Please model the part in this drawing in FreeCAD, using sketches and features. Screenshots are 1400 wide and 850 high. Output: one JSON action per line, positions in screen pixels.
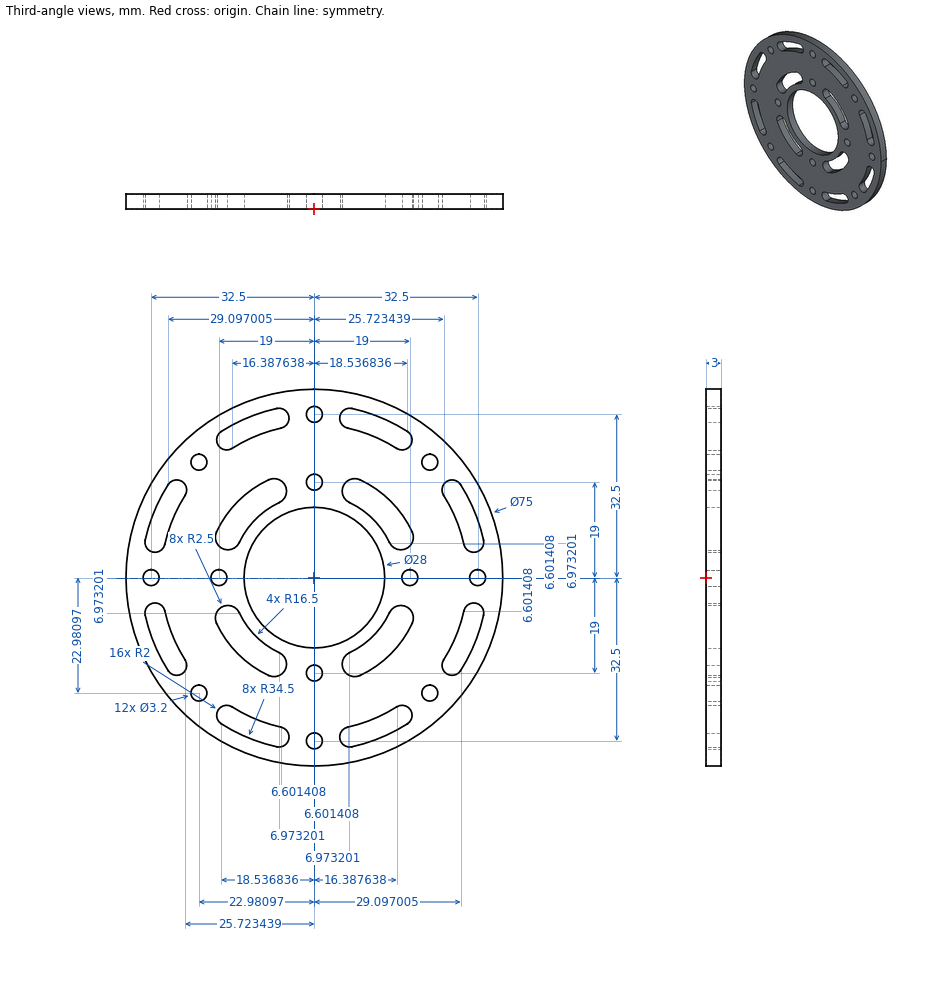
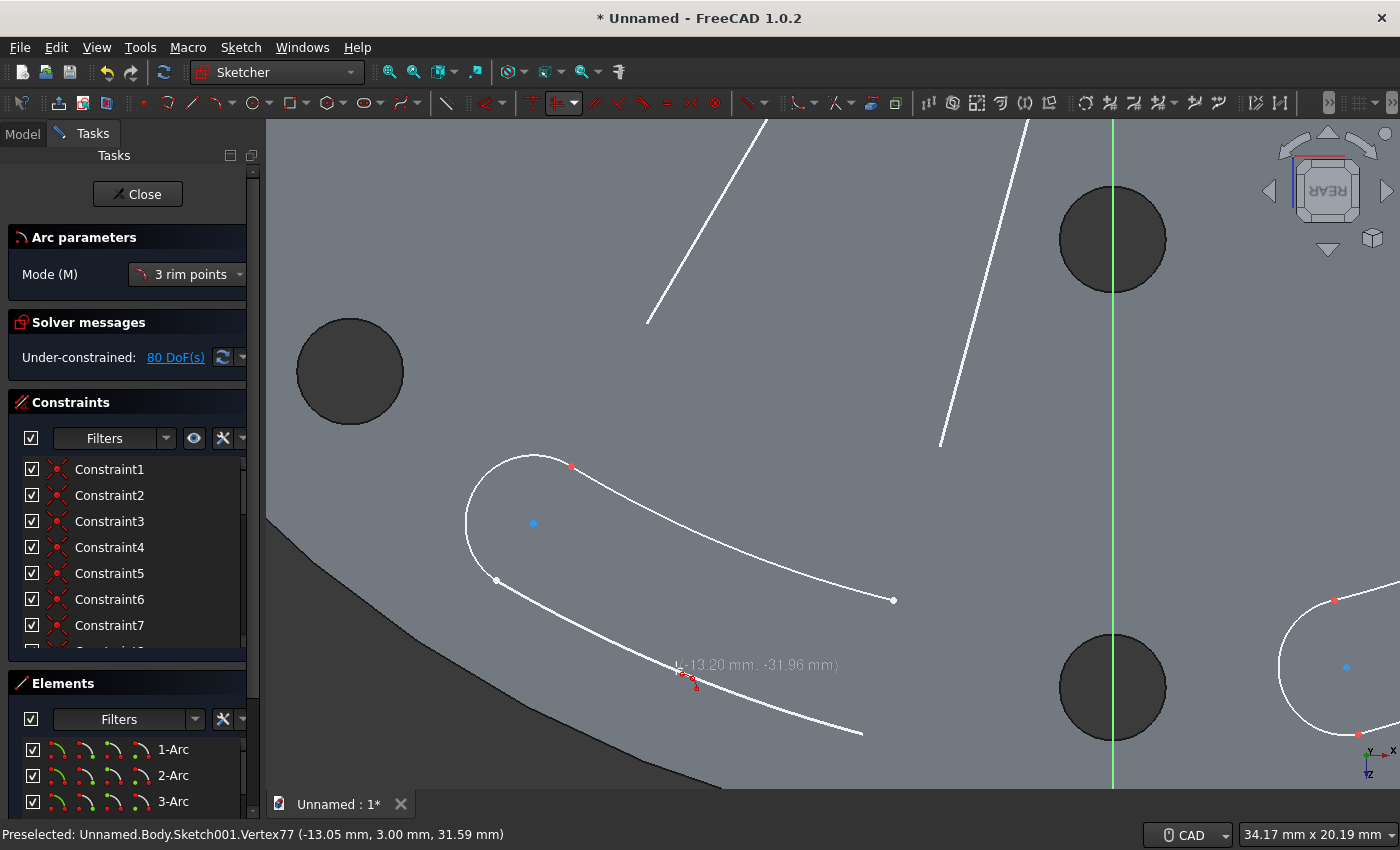
{"action": "left_click", "coordinate": [675, 667]}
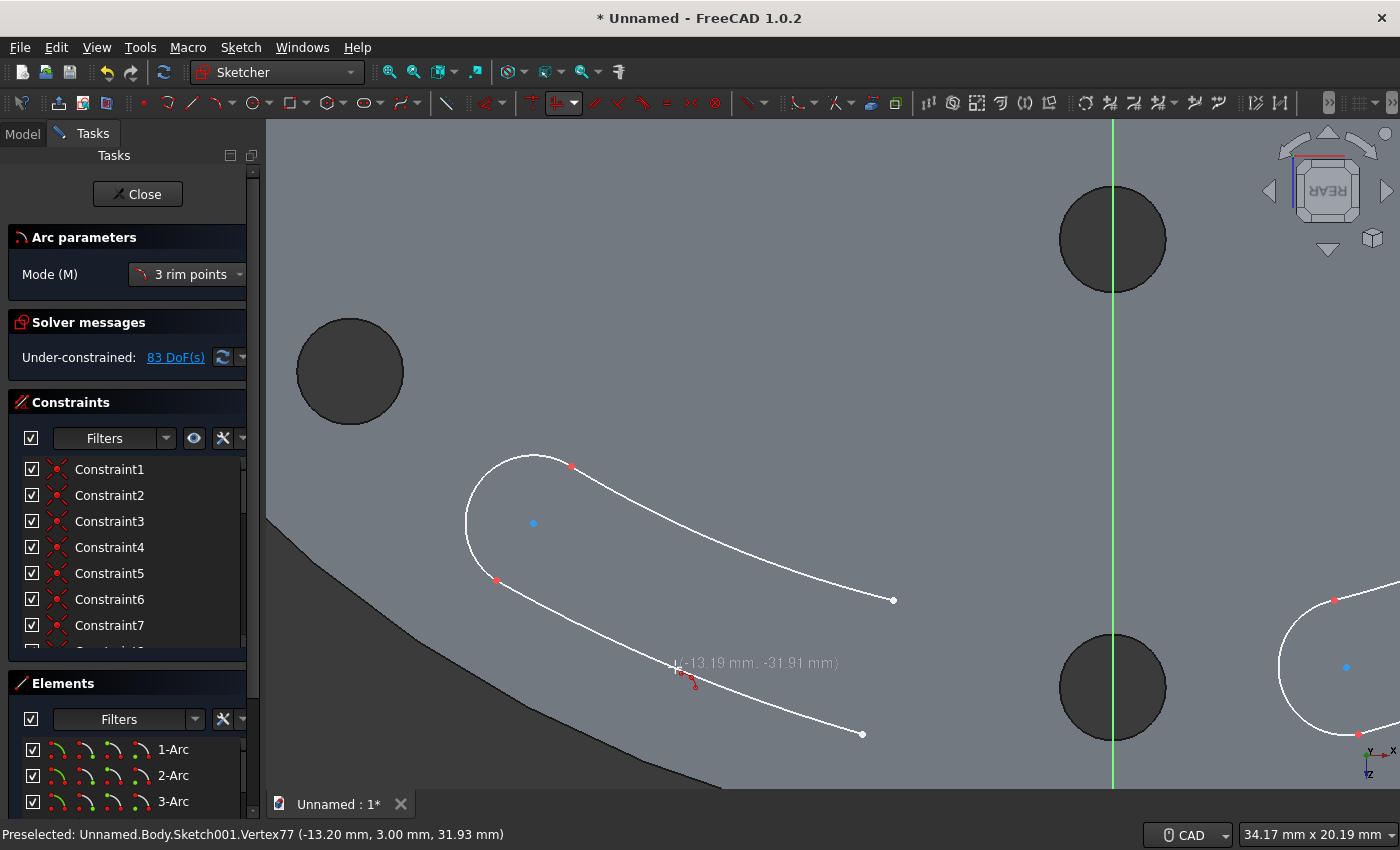
{"action": "scroll", "coordinate": [676, 668], "scroll_direction": "down", "scroll_amount": 8}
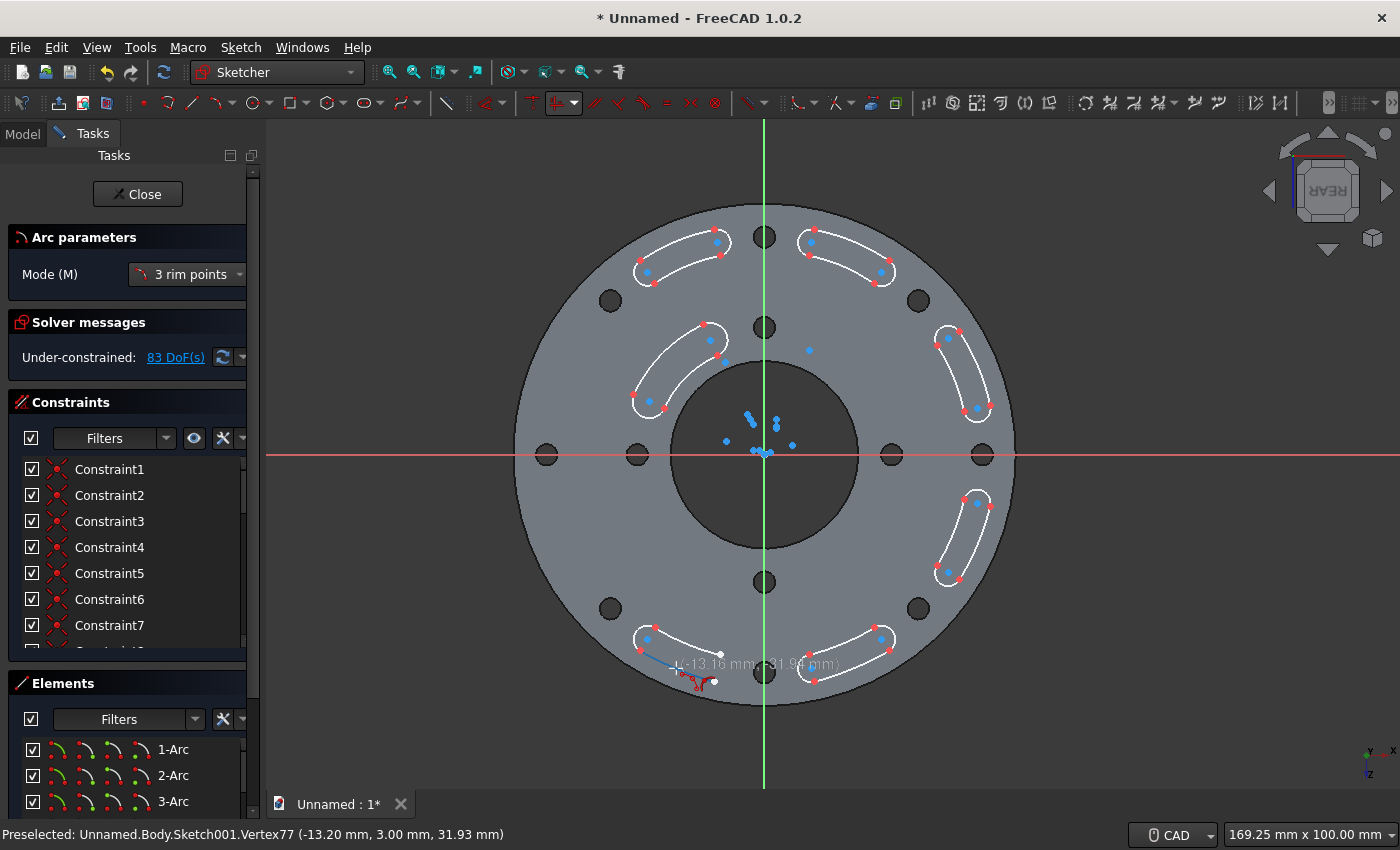
{"action": "left_click", "coordinate": [714, 682]}
{"action": "left_click", "coordinate": [720, 655]}
{"action": "left_click", "coordinate": [730, 670]}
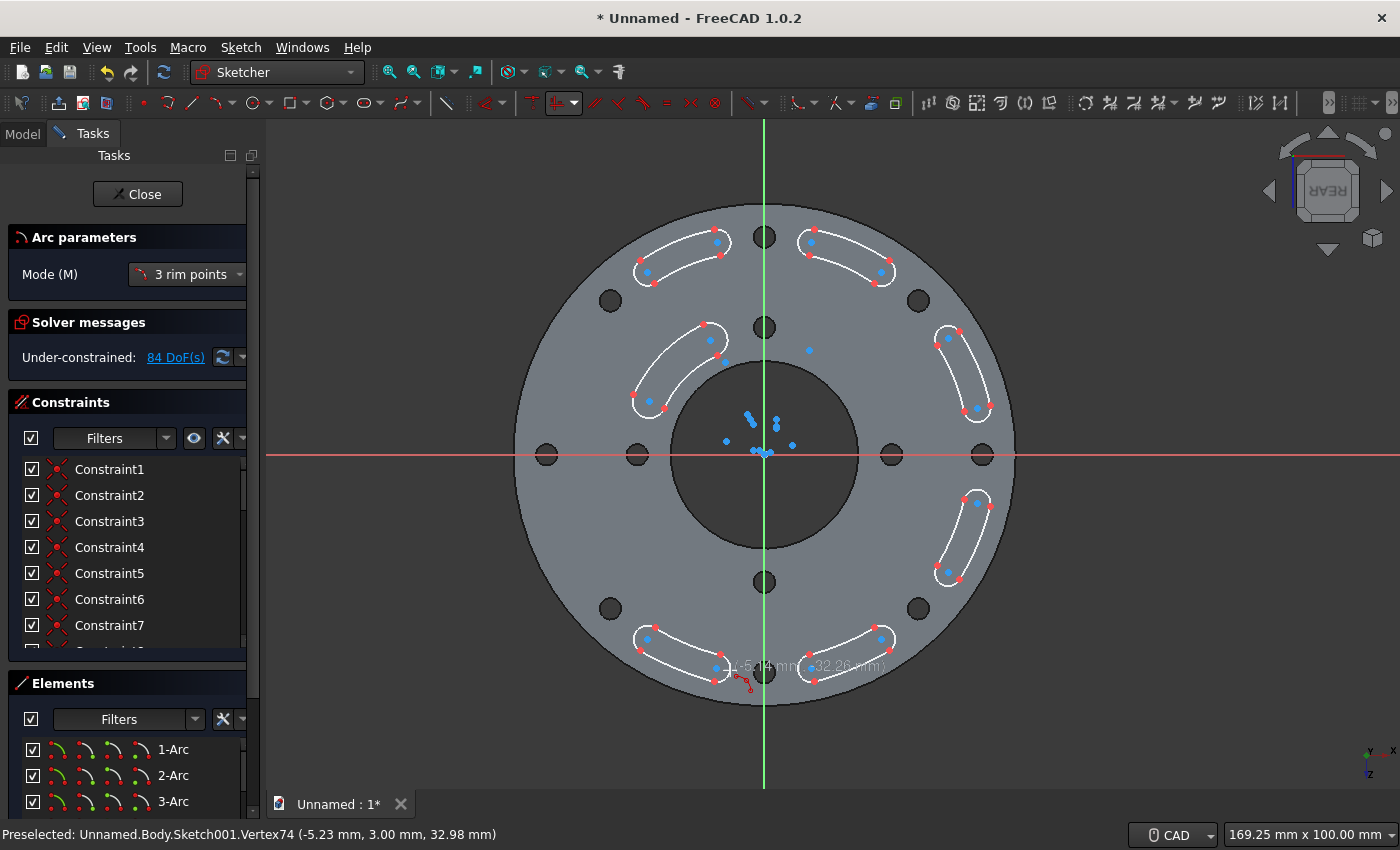
{"action": "left_click", "coordinate": [565, 499]}
{"action": "left_click", "coordinate": [539, 505]}
{"action": "left_click", "coordinate": [549, 489]}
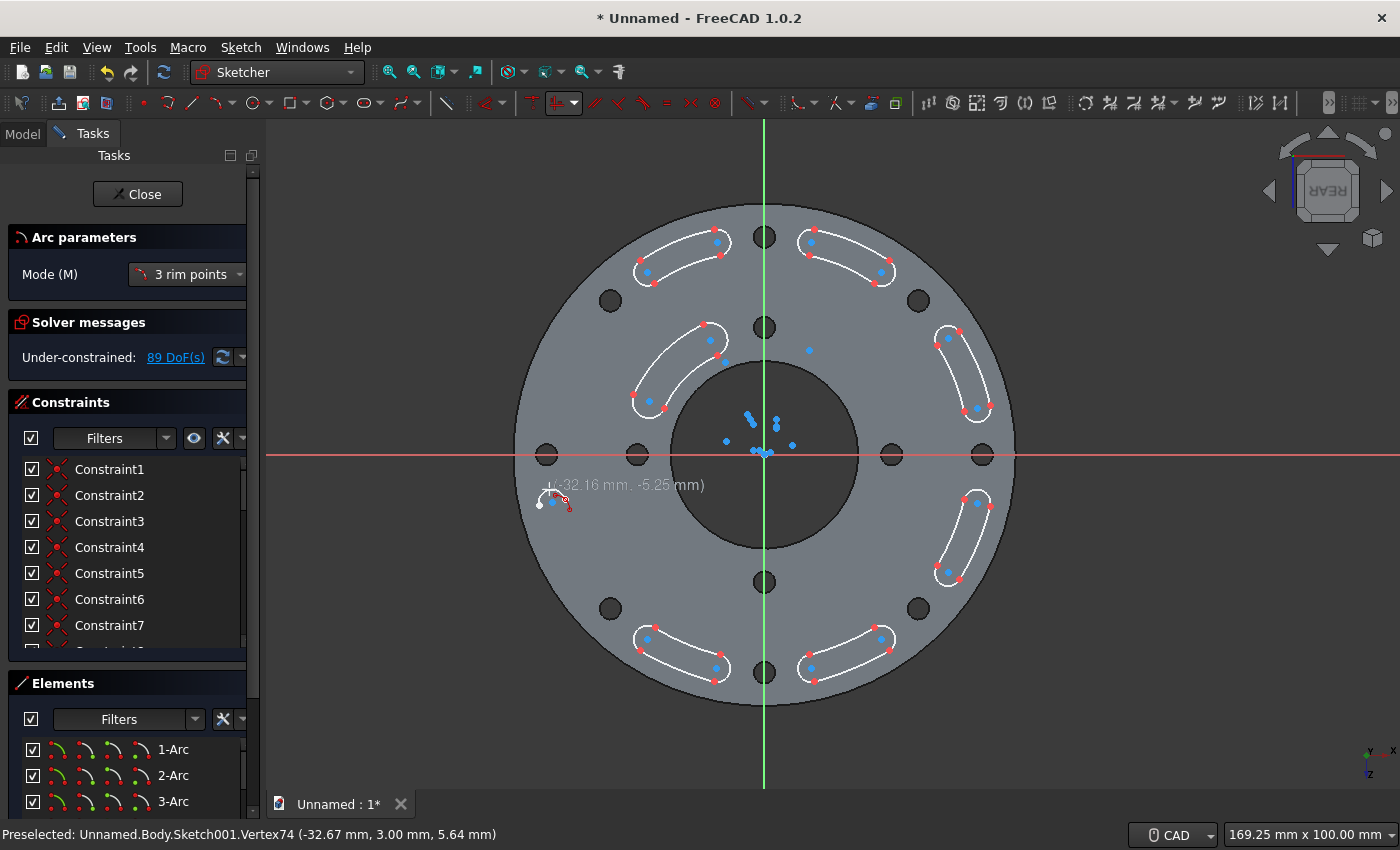
{"action": "left_click", "coordinate": [539, 506]}
{"action": "left_click", "coordinate": [570, 579]}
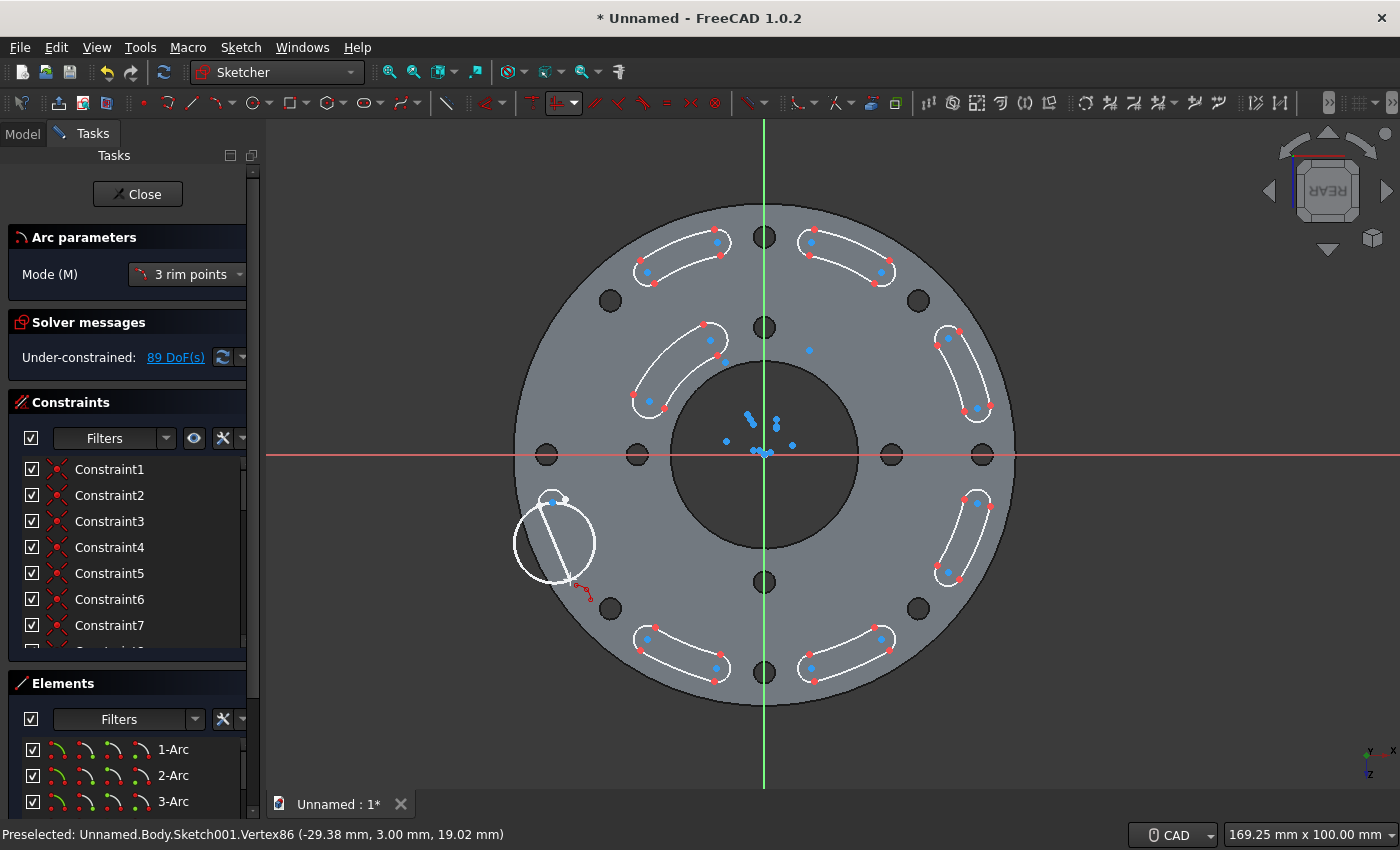
{"action": "scroll", "coordinate": [551, 543], "scroll_direction": "up", "scroll_amount": 8}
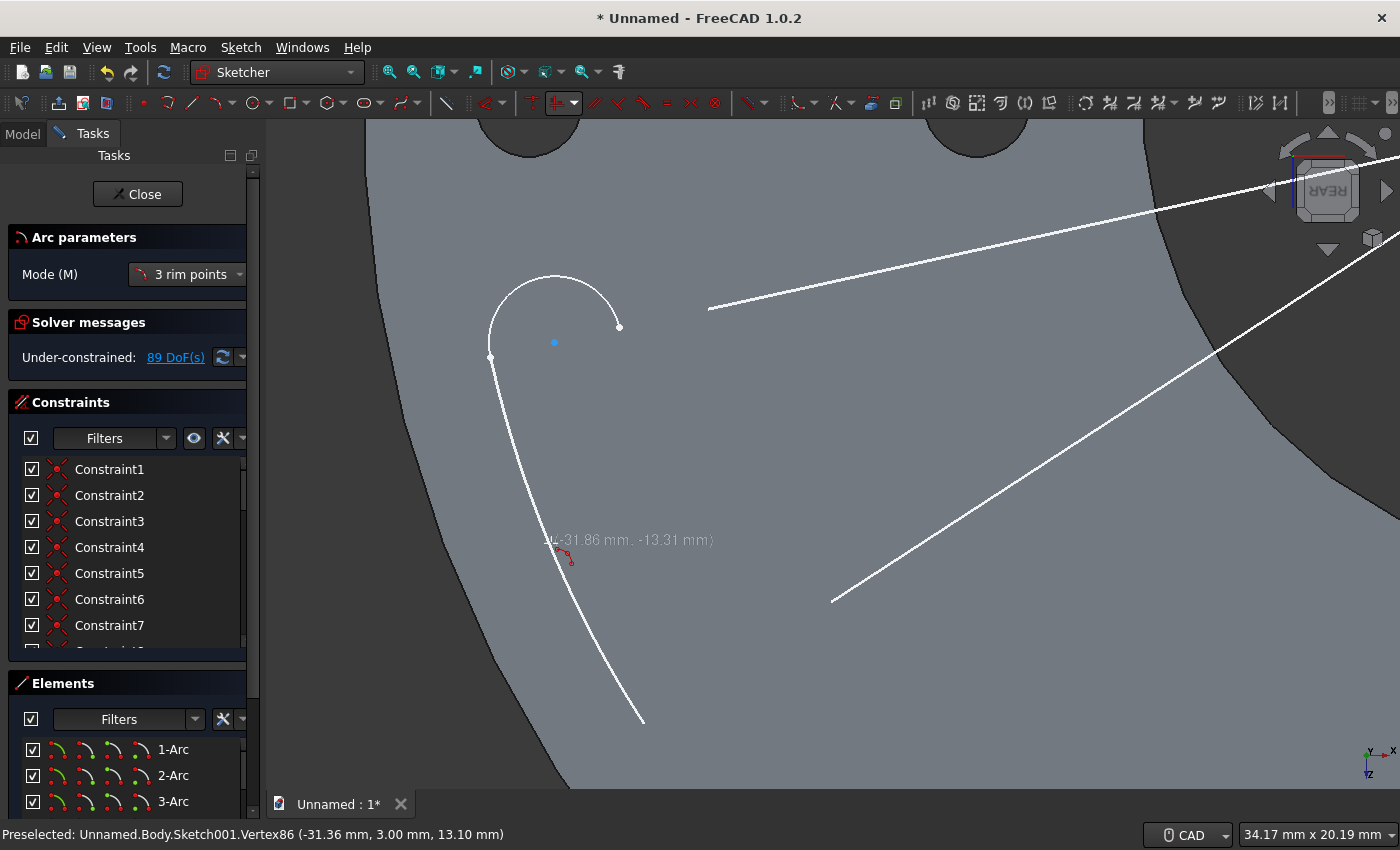
{"action": "left_click", "coordinate": [550, 542]}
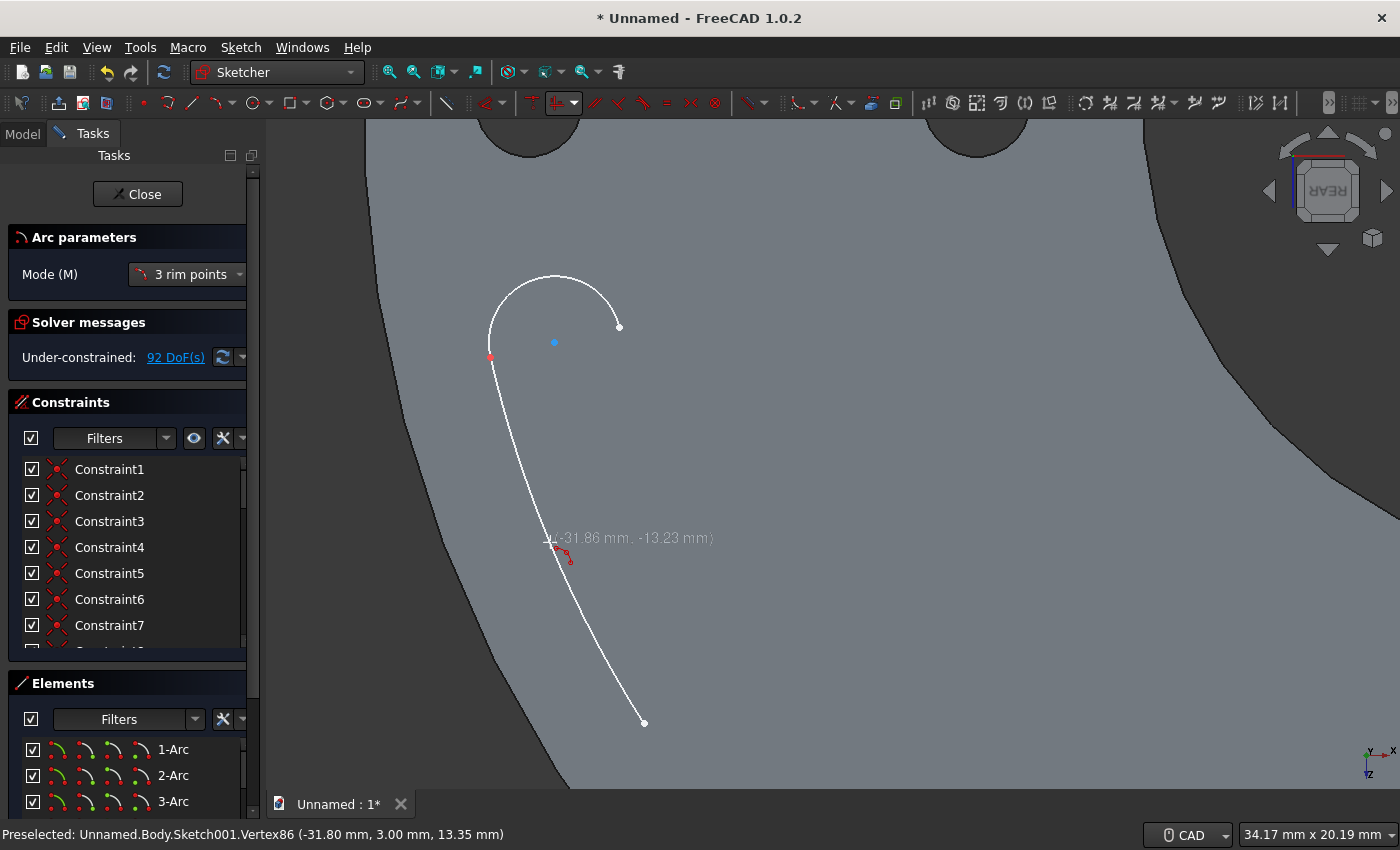
{"action": "scroll", "coordinate": [551, 543], "scroll_direction": "down", "scroll_amount": 8}